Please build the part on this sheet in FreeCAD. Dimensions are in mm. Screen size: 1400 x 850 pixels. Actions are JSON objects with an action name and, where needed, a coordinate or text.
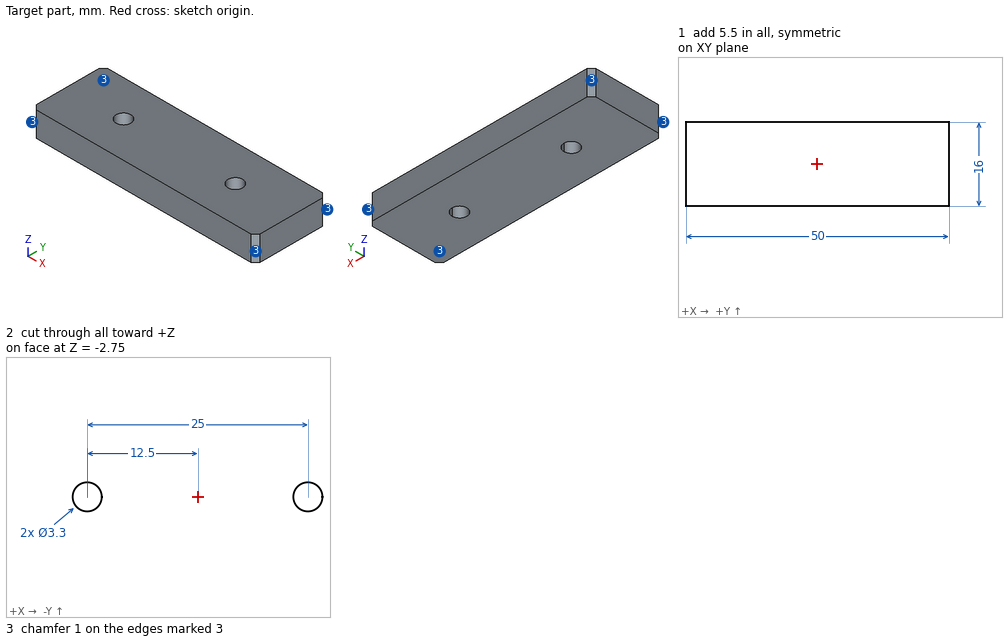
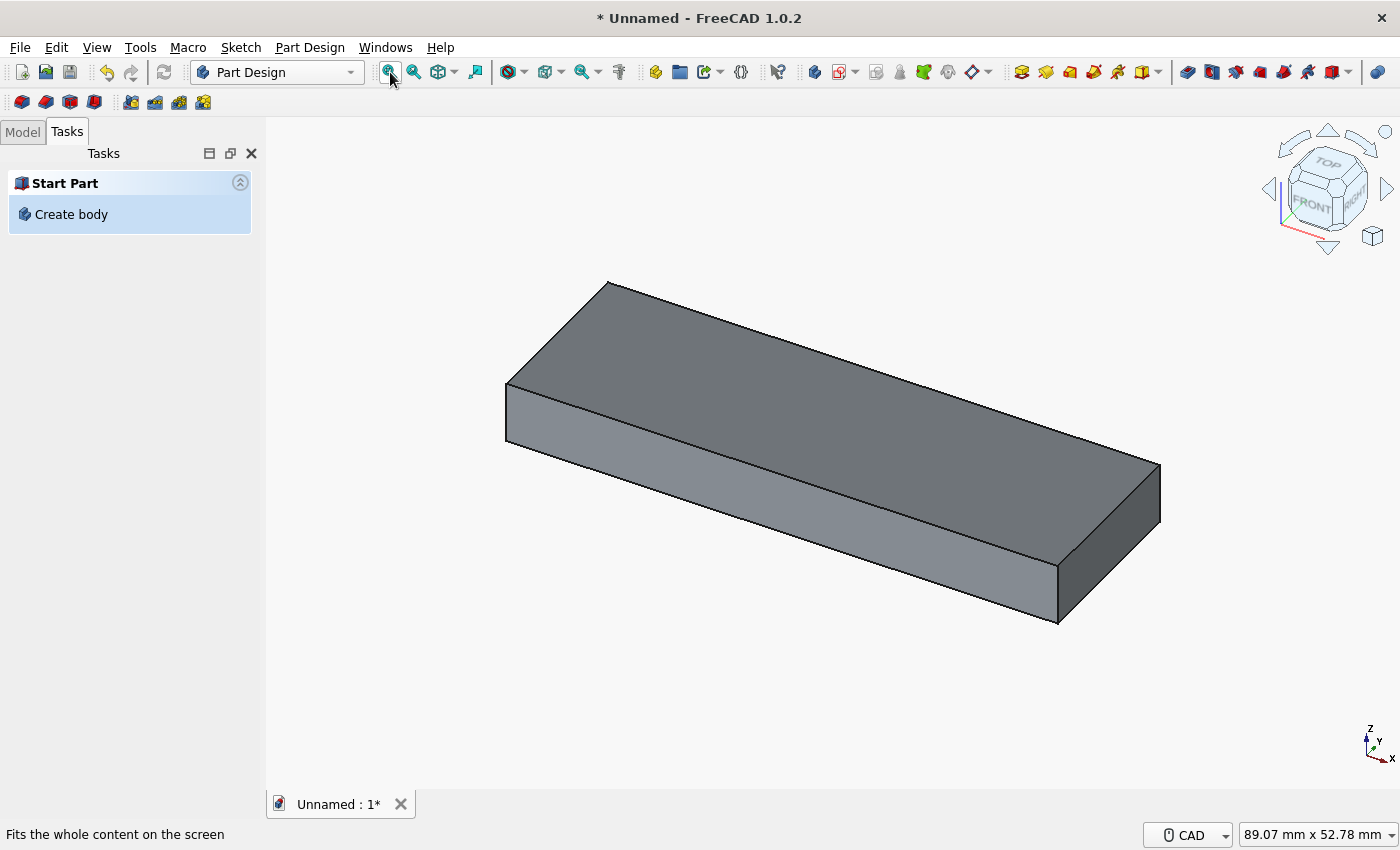
{"action": "key", "text": "5"}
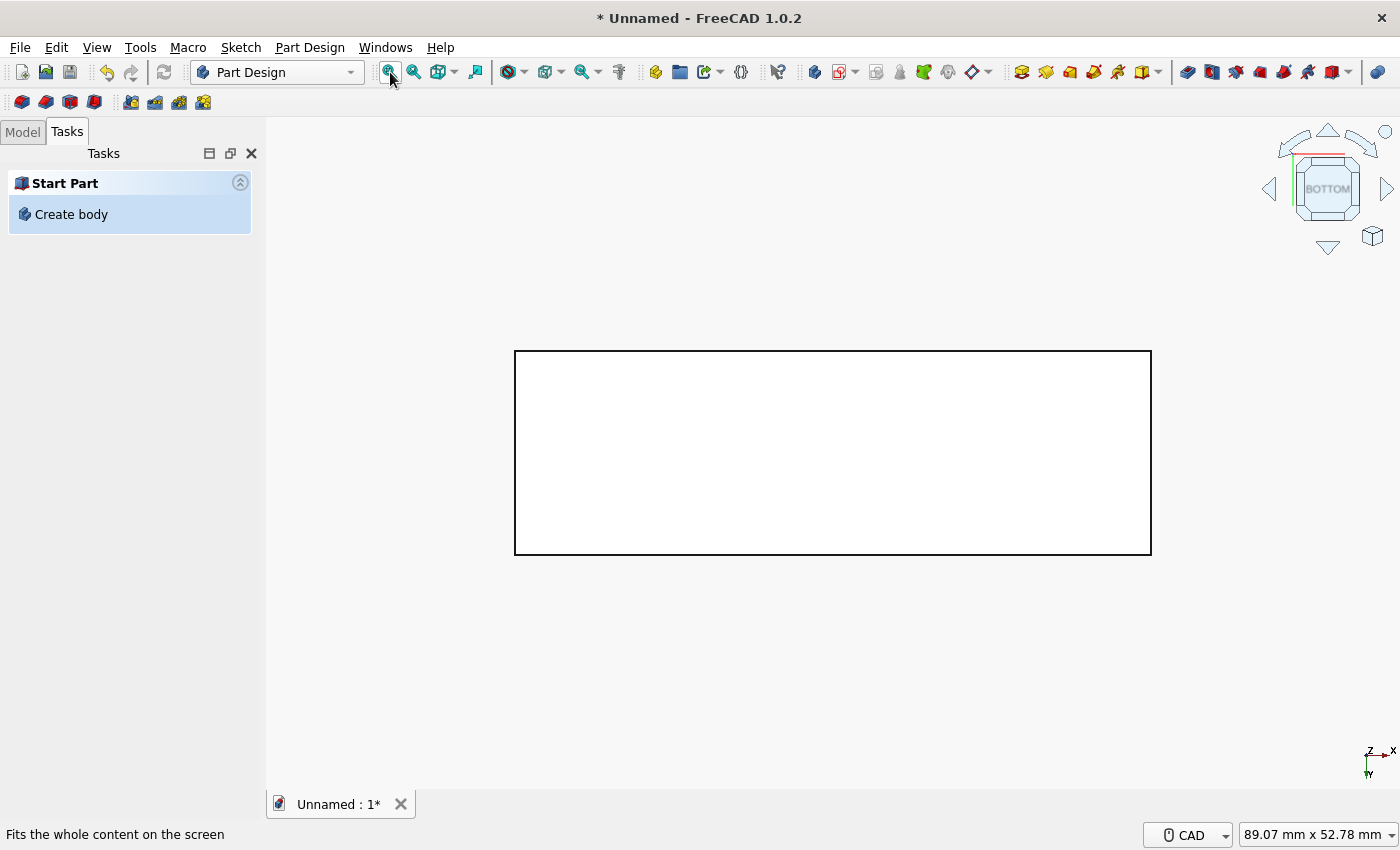
{"action": "left_click", "coordinate": [1015, 452]}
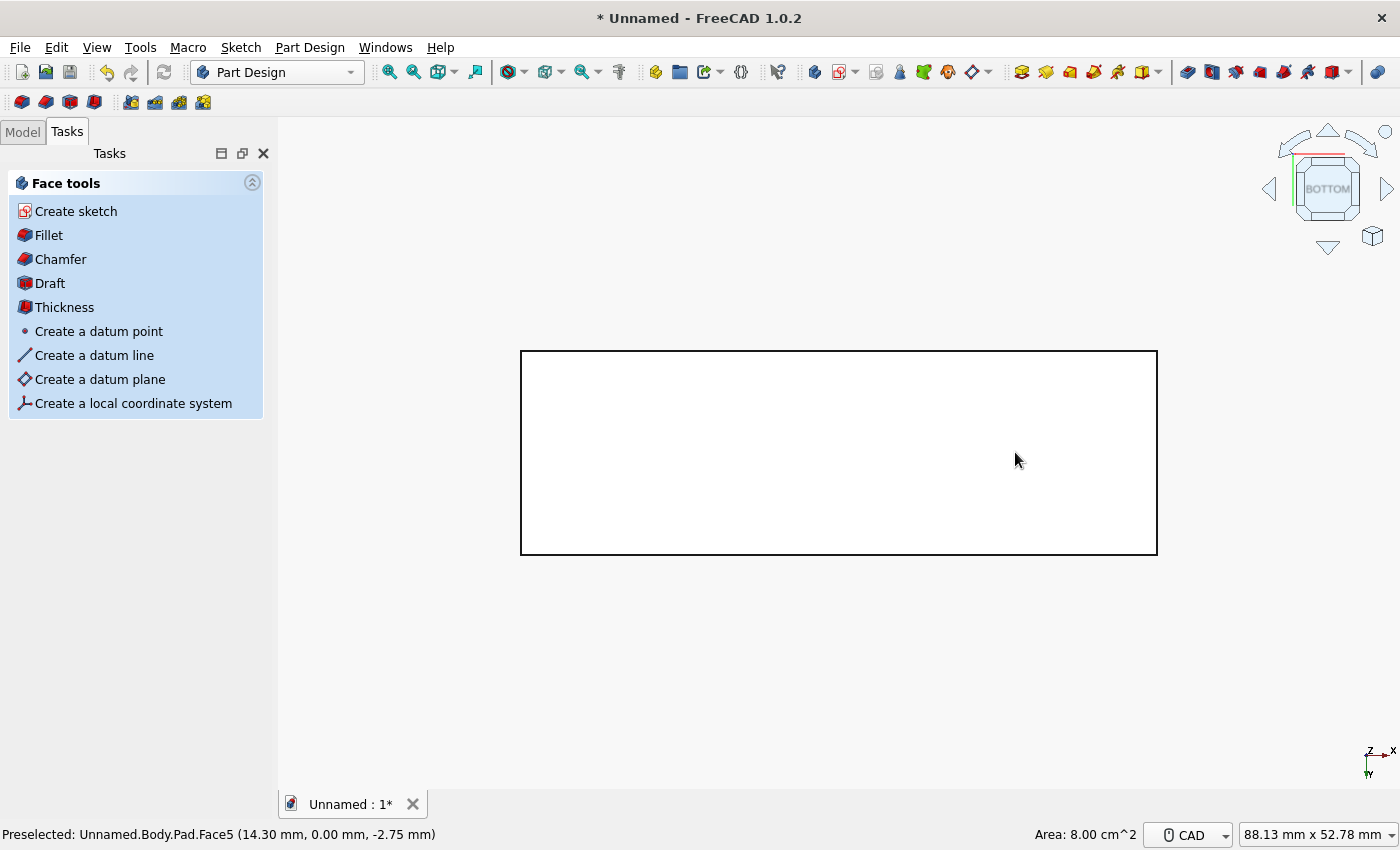
{"action": "left_click", "coordinate": [840, 72]}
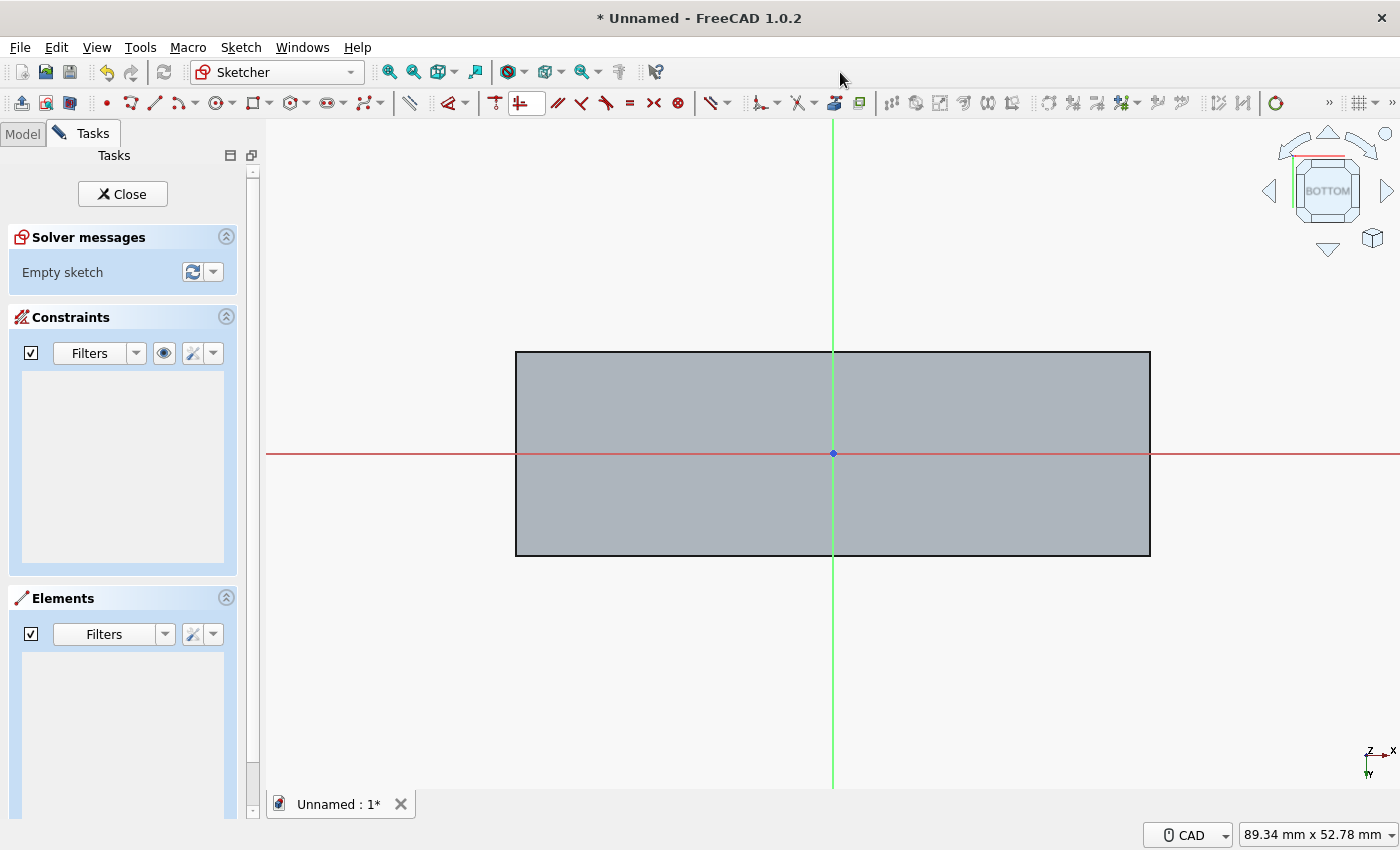
{"action": "scroll", "coordinate": [916, 454], "scroll_direction": "up", "scroll_amount": 3}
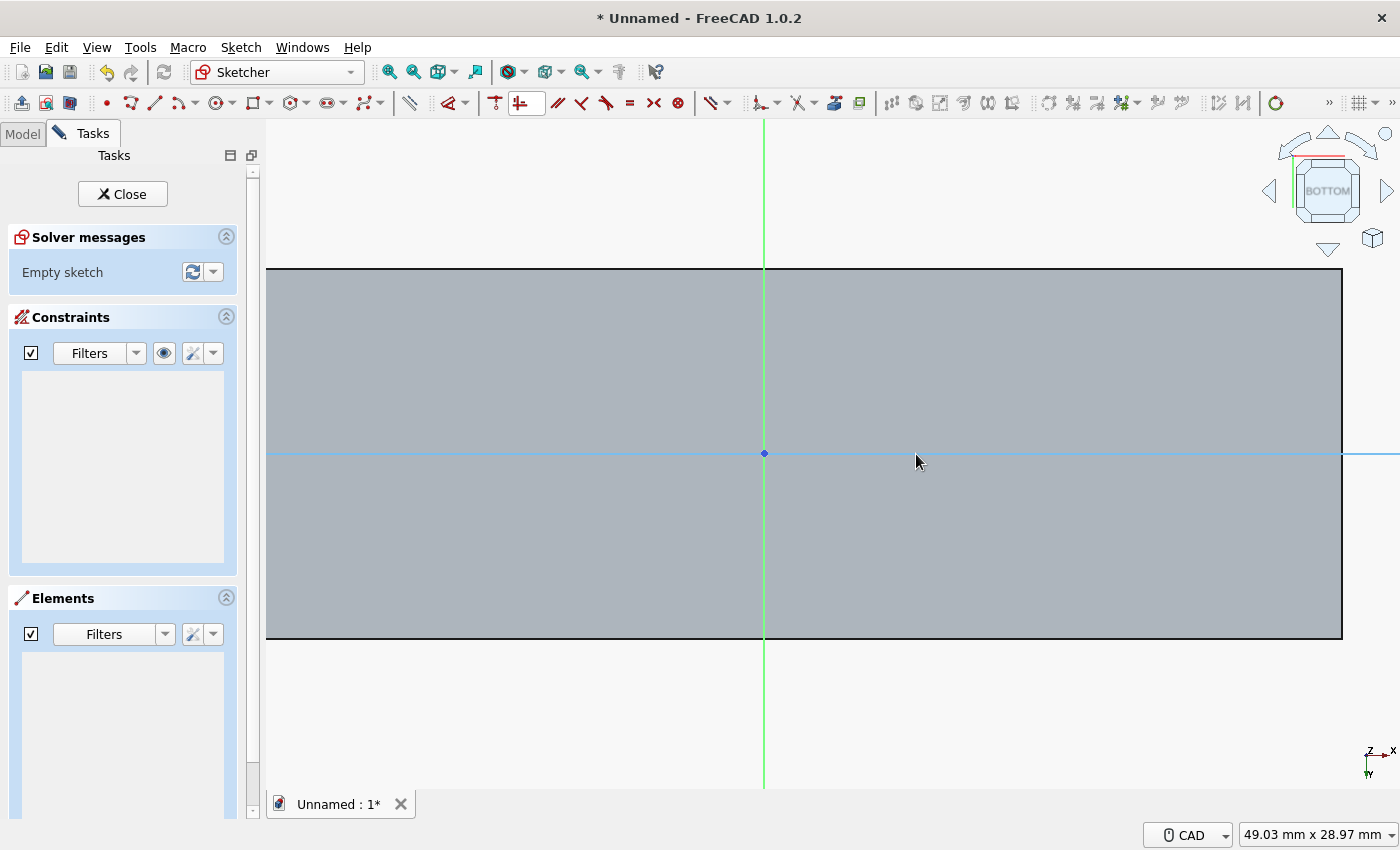
{"action": "left_click", "coordinate": [216, 104]}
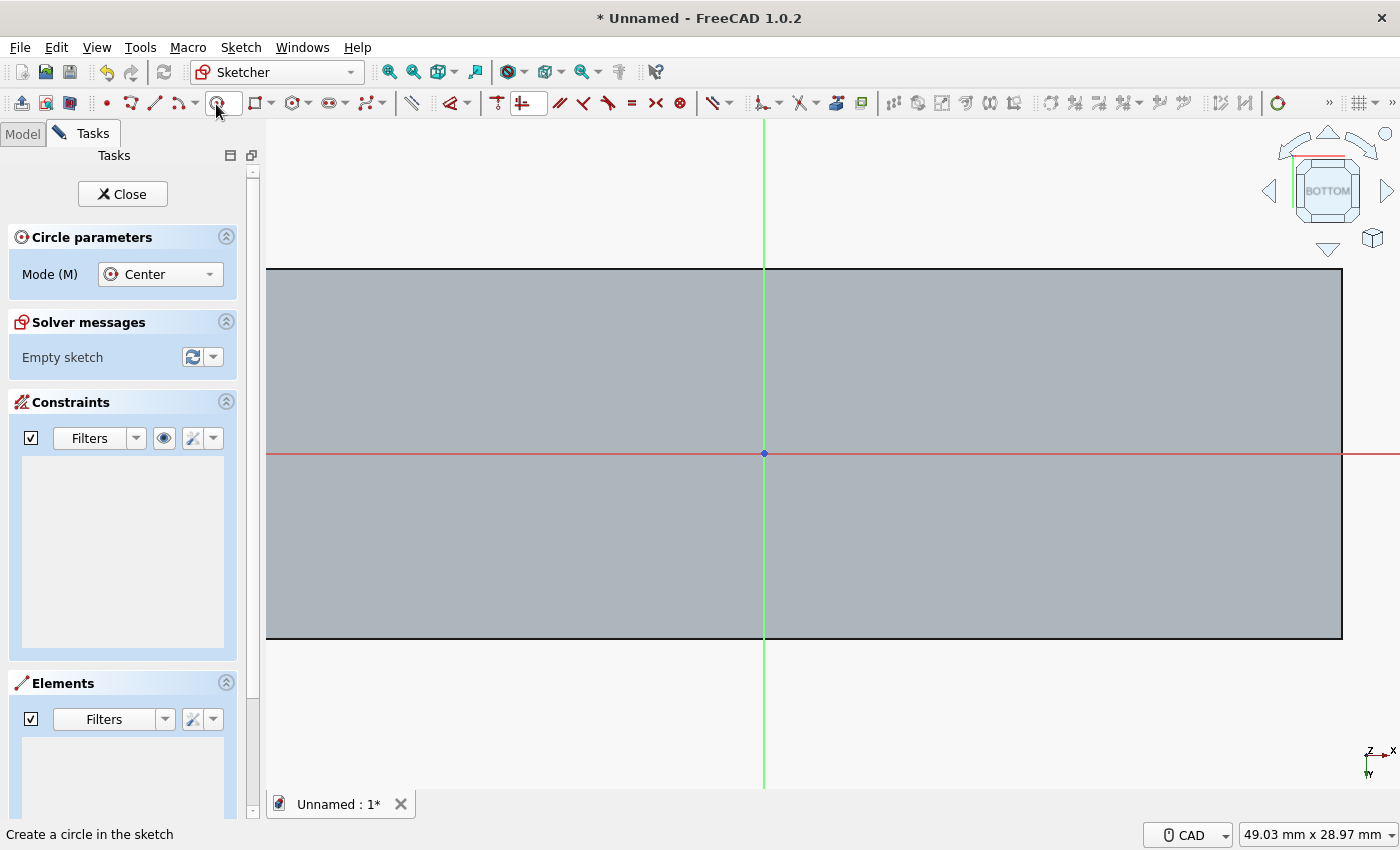
{"action": "left_click", "coordinate": [475, 454]}
{"action": "left_click", "coordinate": [502, 427]}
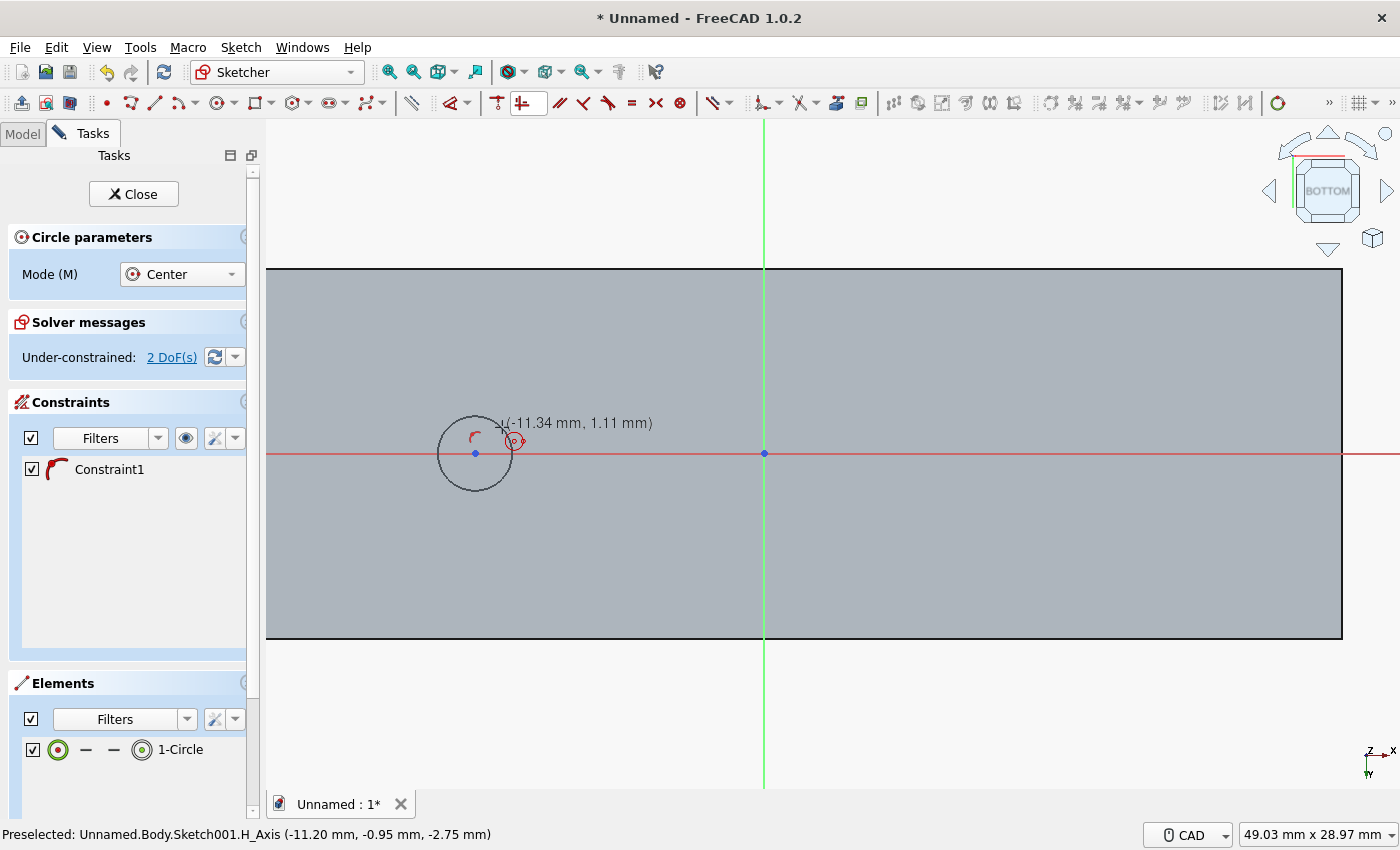
{"action": "left_click", "coordinate": [1053, 454]}
{"action": "left_click", "coordinate": [1080, 427]}
{"action": "key", "text": "Escape"}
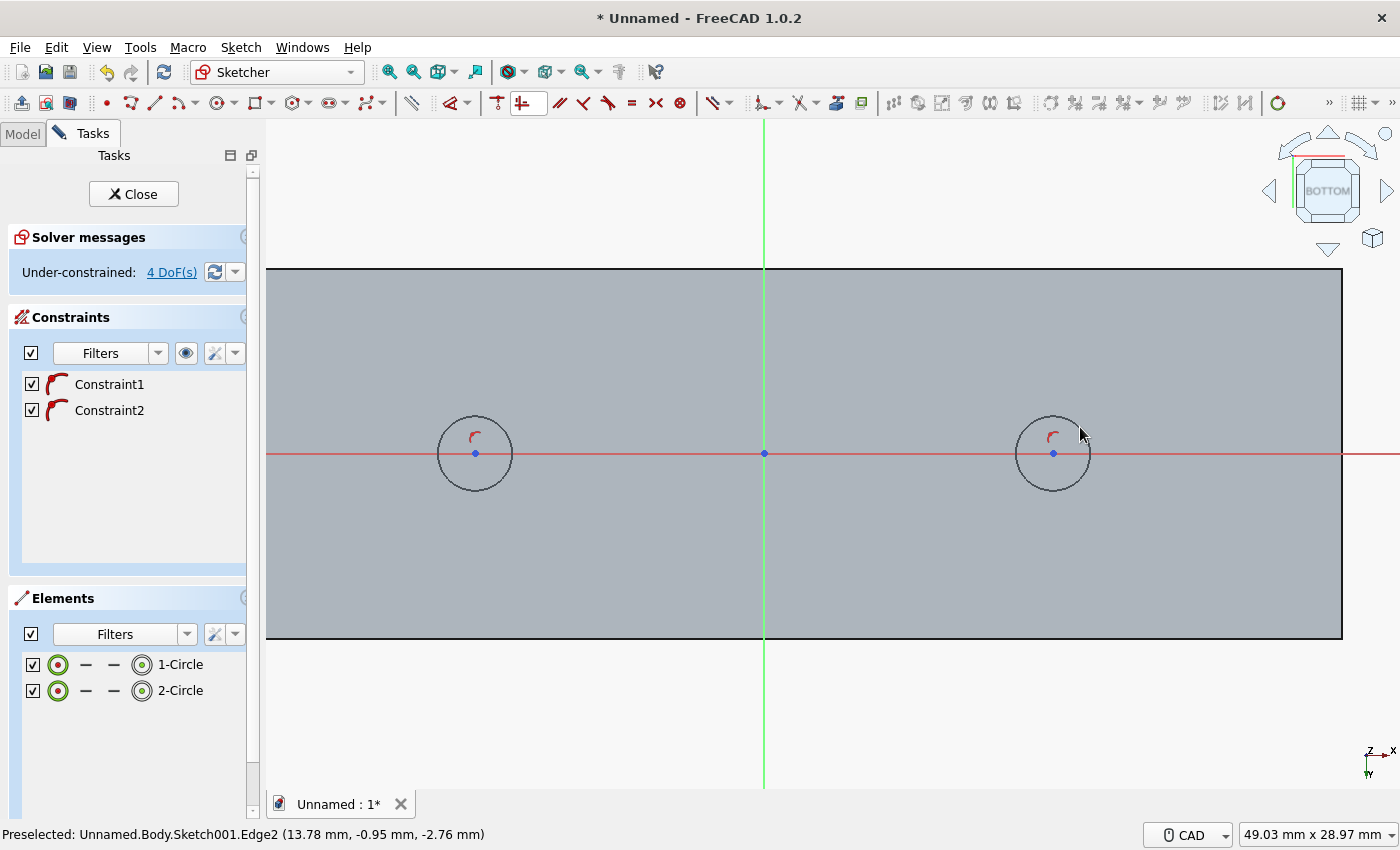
{"action": "left_click", "coordinate": [501, 427]}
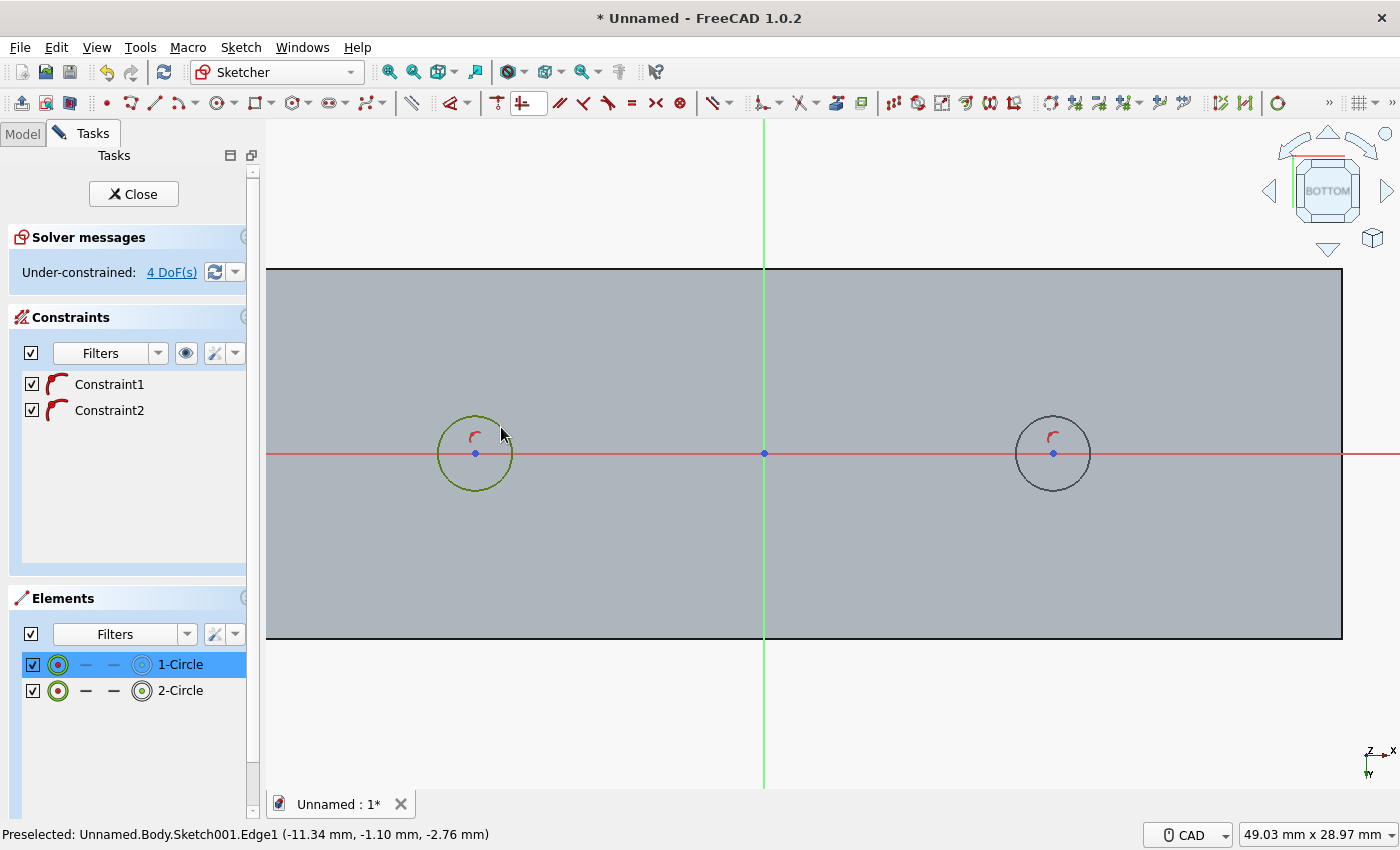
{"action": "left_click", "coordinate": [1079, 427]}